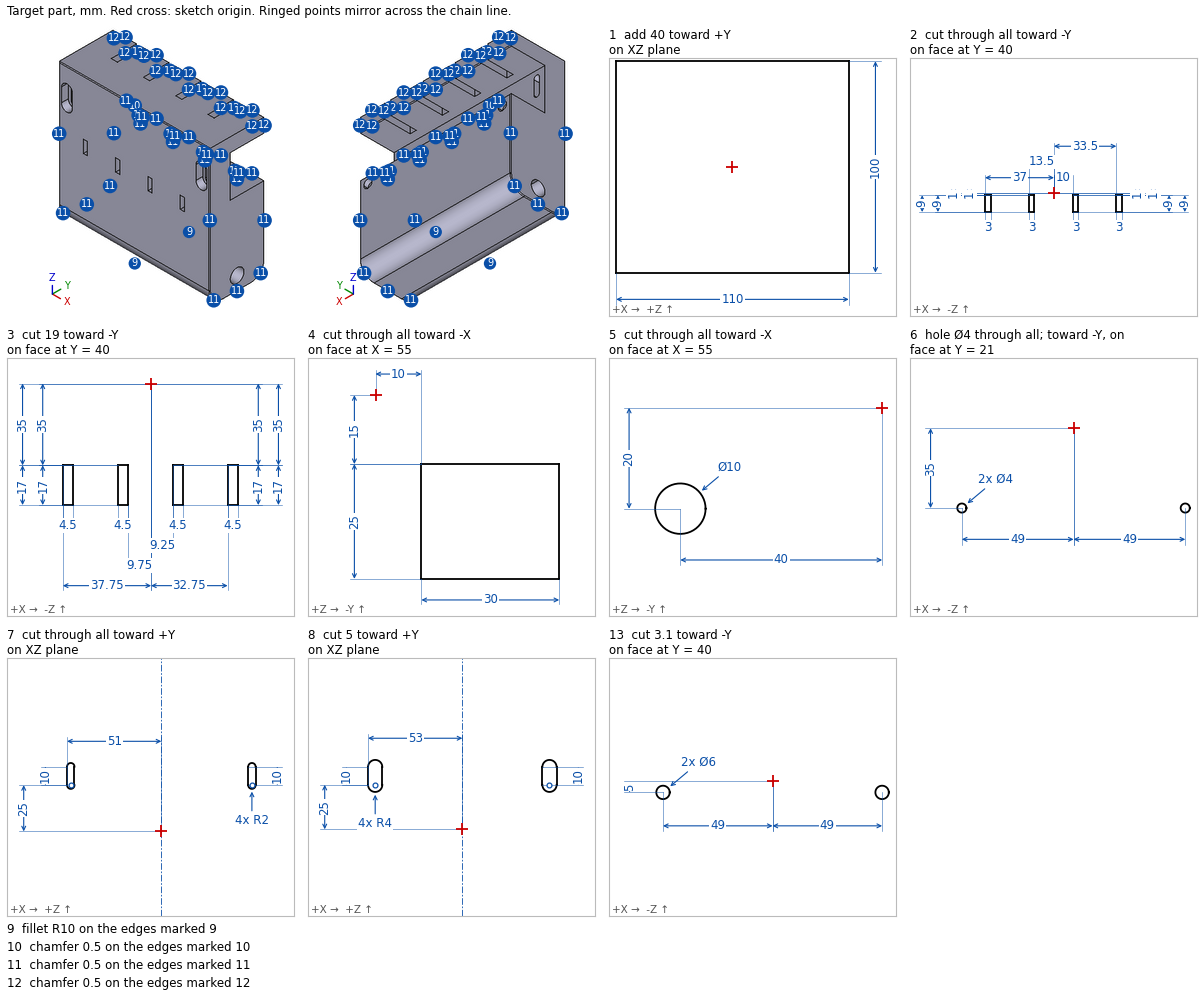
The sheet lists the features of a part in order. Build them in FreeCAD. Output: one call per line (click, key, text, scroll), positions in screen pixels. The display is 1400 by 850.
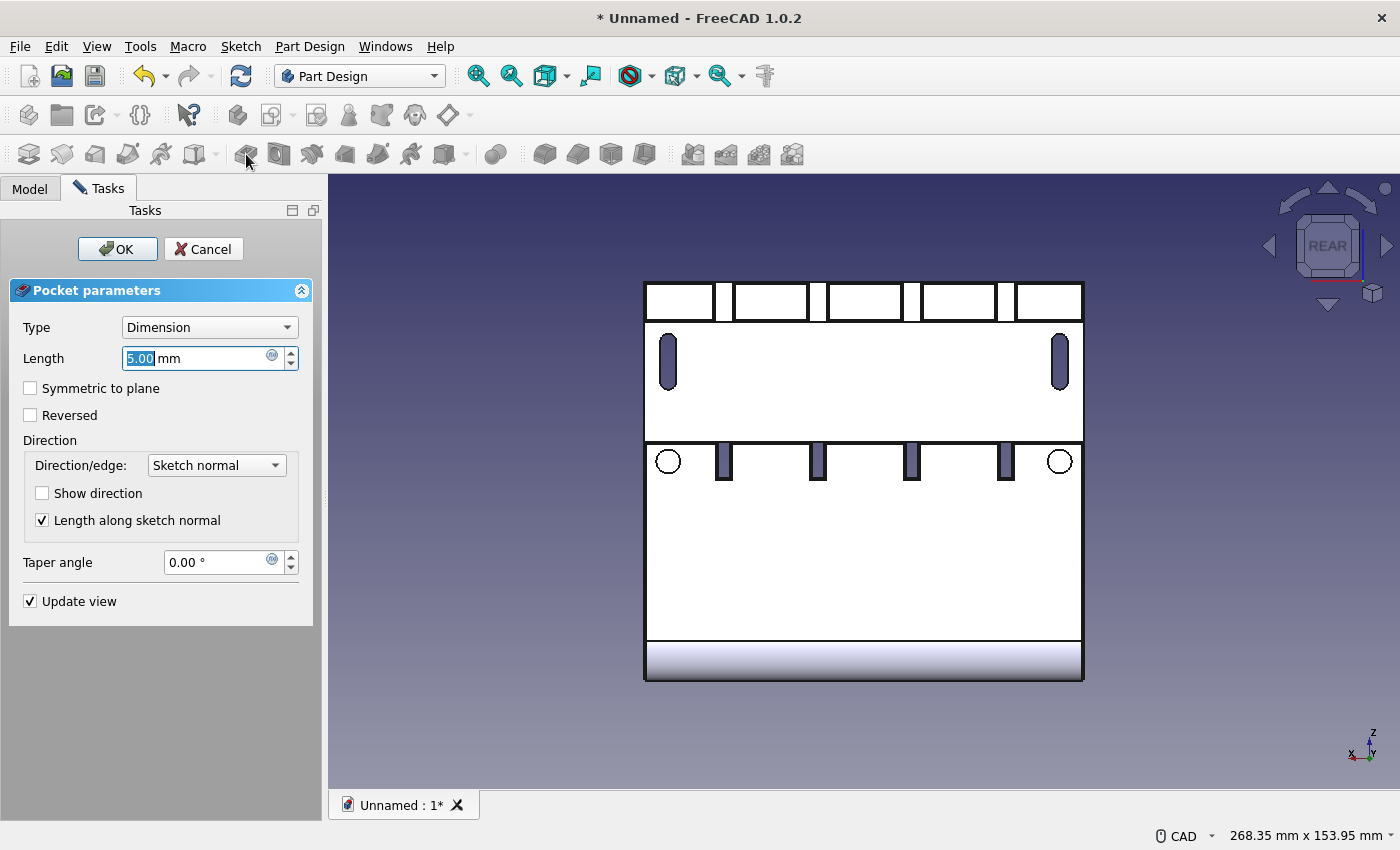
text(3.1)
key(Tab)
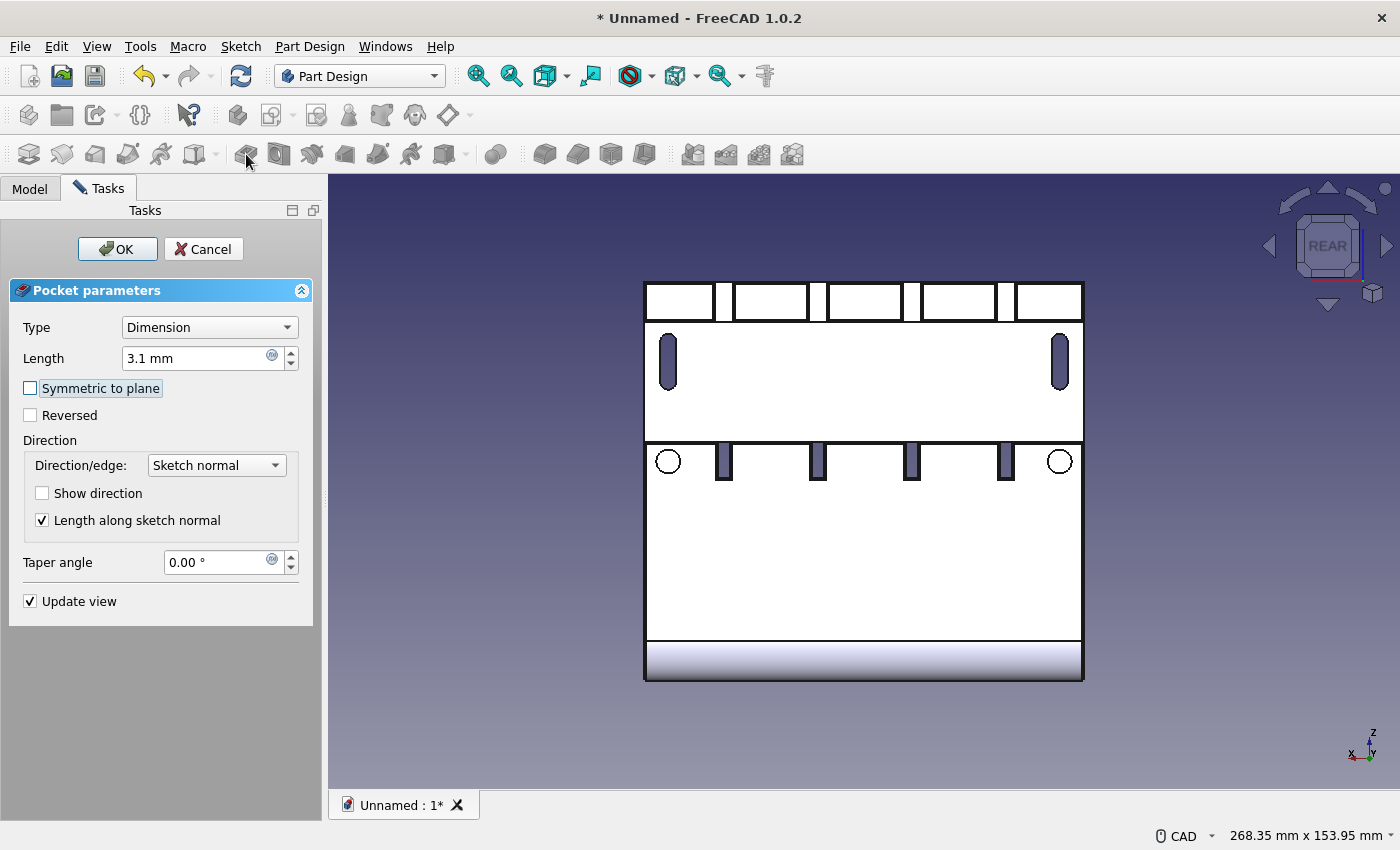
click(118, 249)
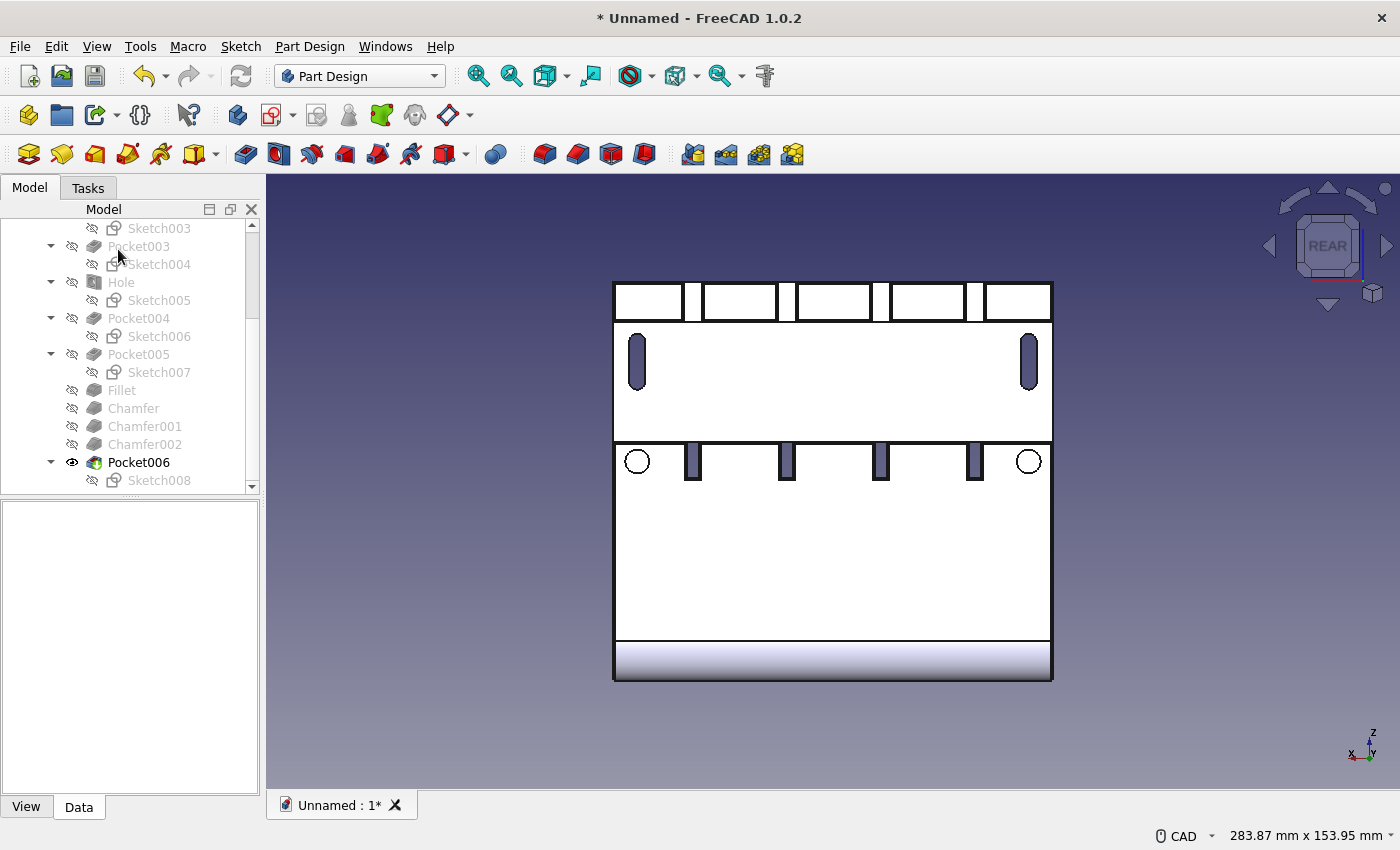
key(0)